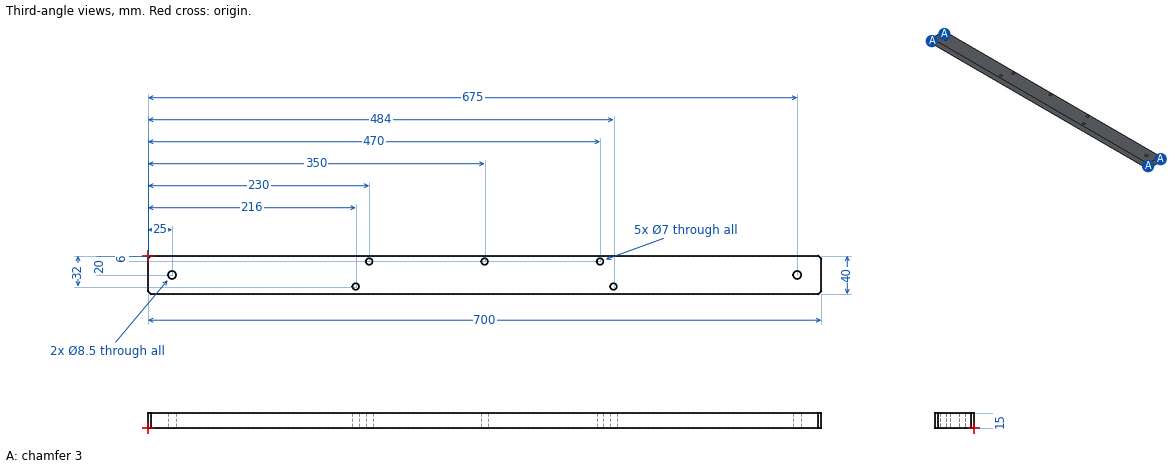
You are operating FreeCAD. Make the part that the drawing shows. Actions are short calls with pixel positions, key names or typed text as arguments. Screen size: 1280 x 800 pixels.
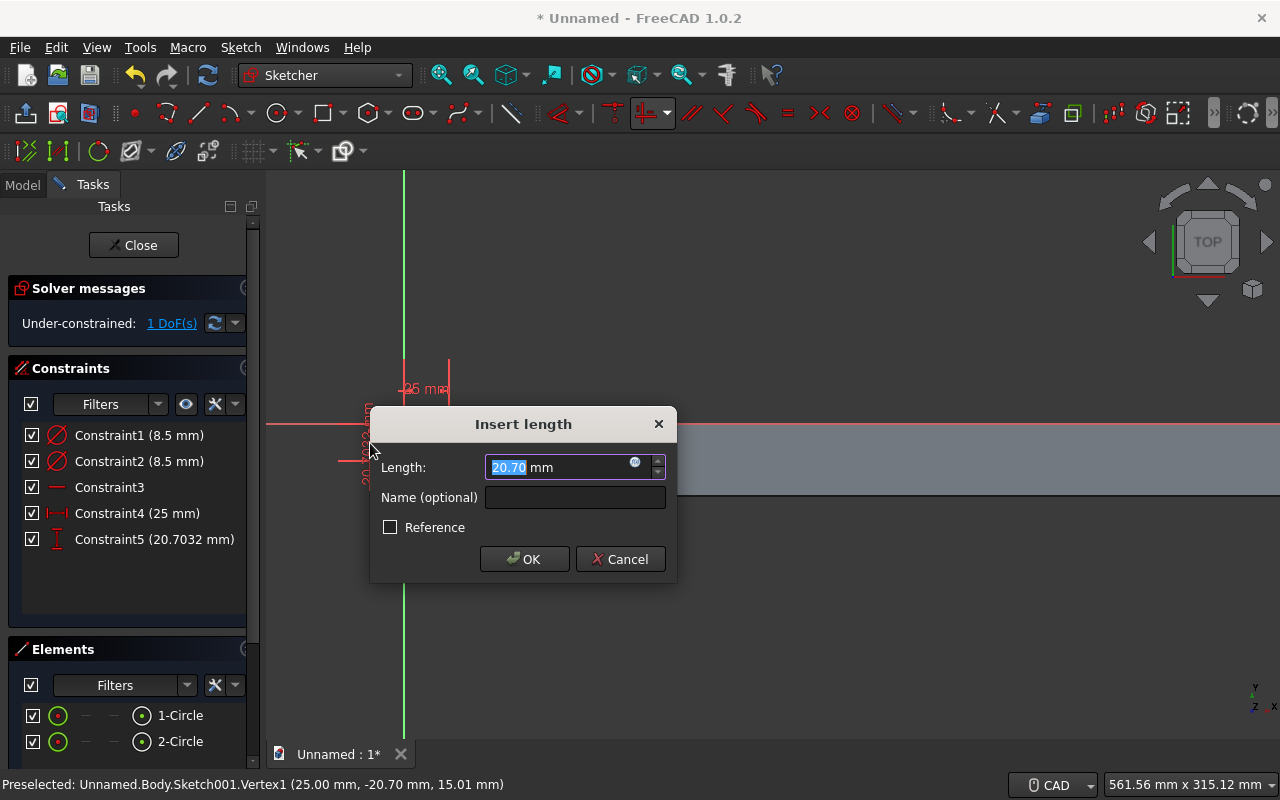
text(20)
key(Return)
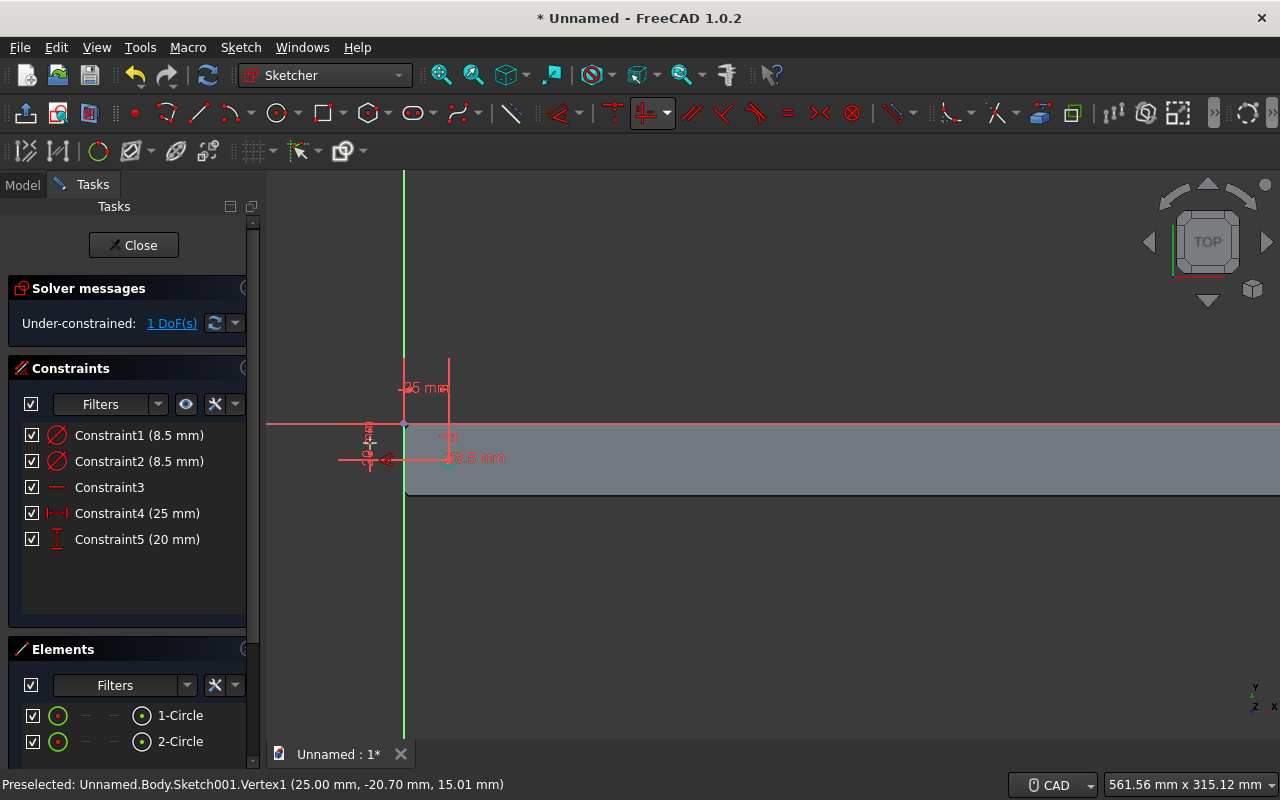
scroll(450, 462, down, 4)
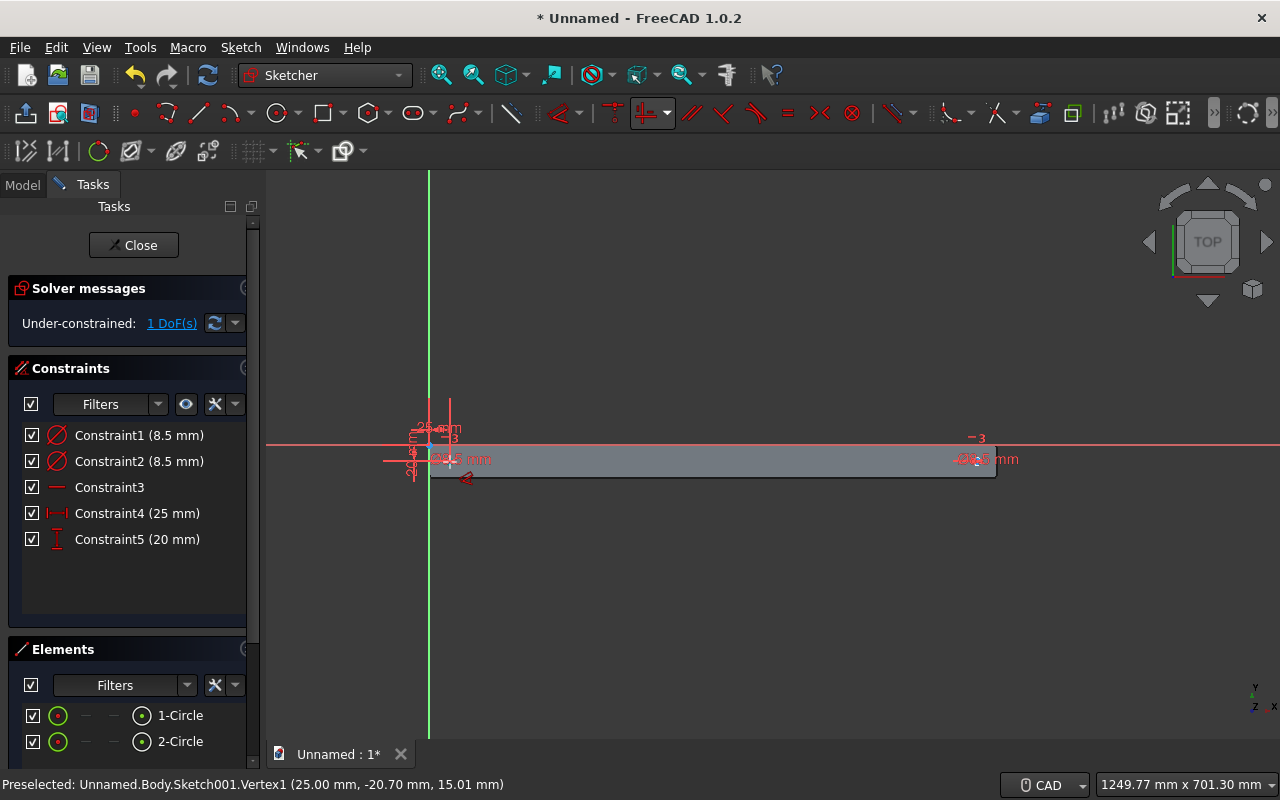
click(977, 461)
click(703, 411)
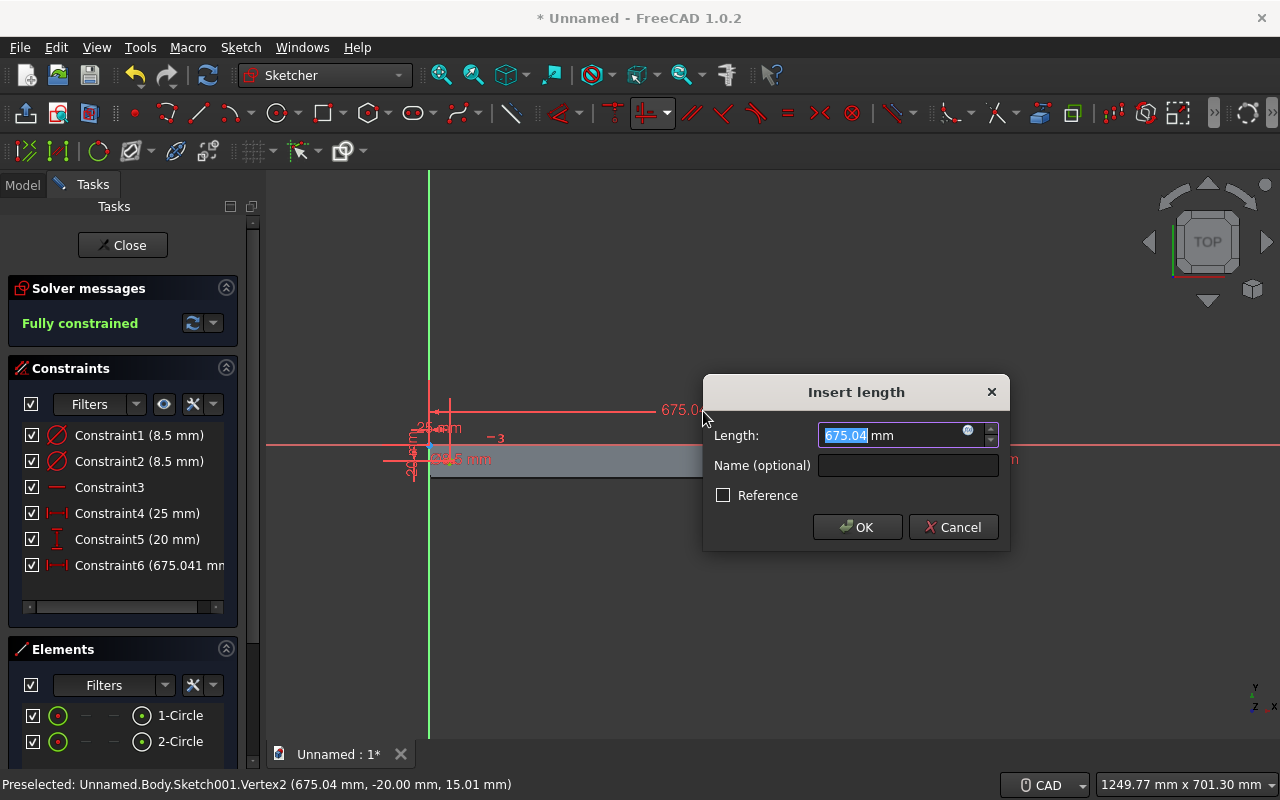
text(675)
key(Return)
key(Escape)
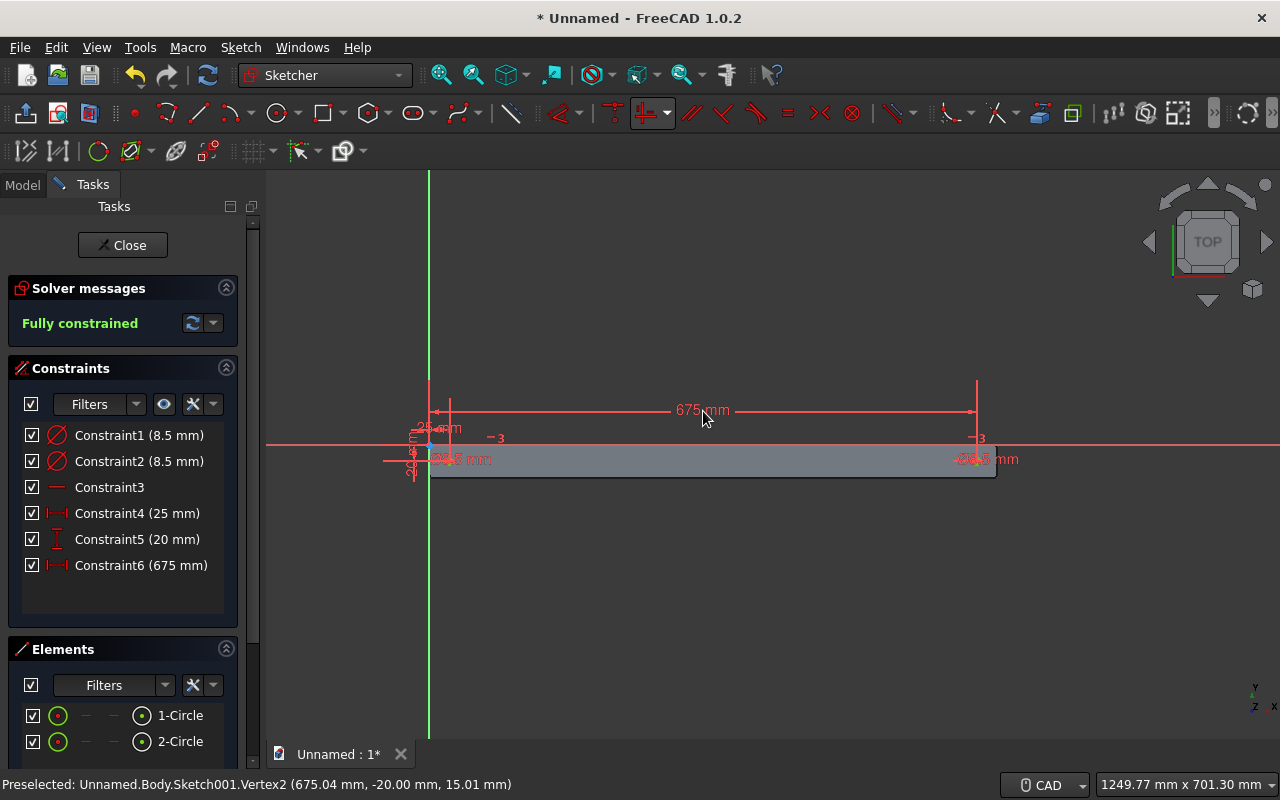
click(123, 245)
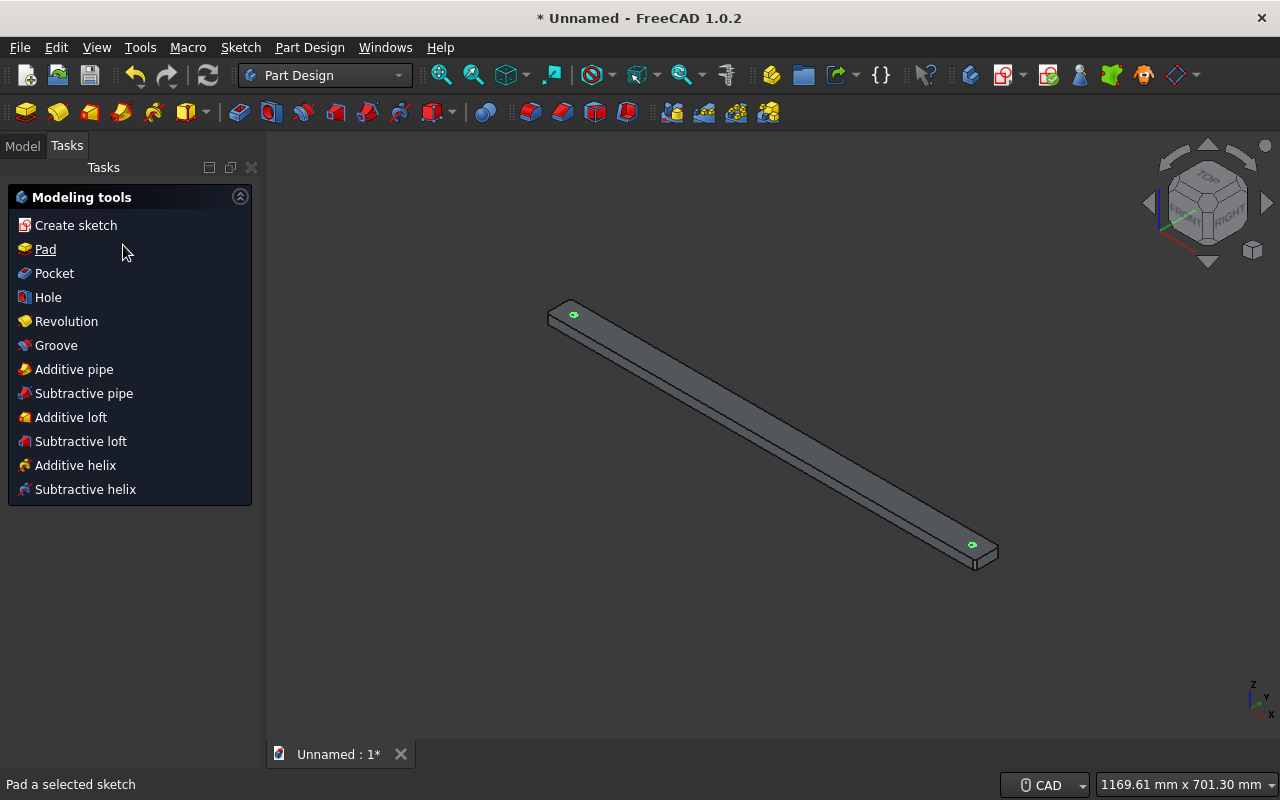
click(272, 112)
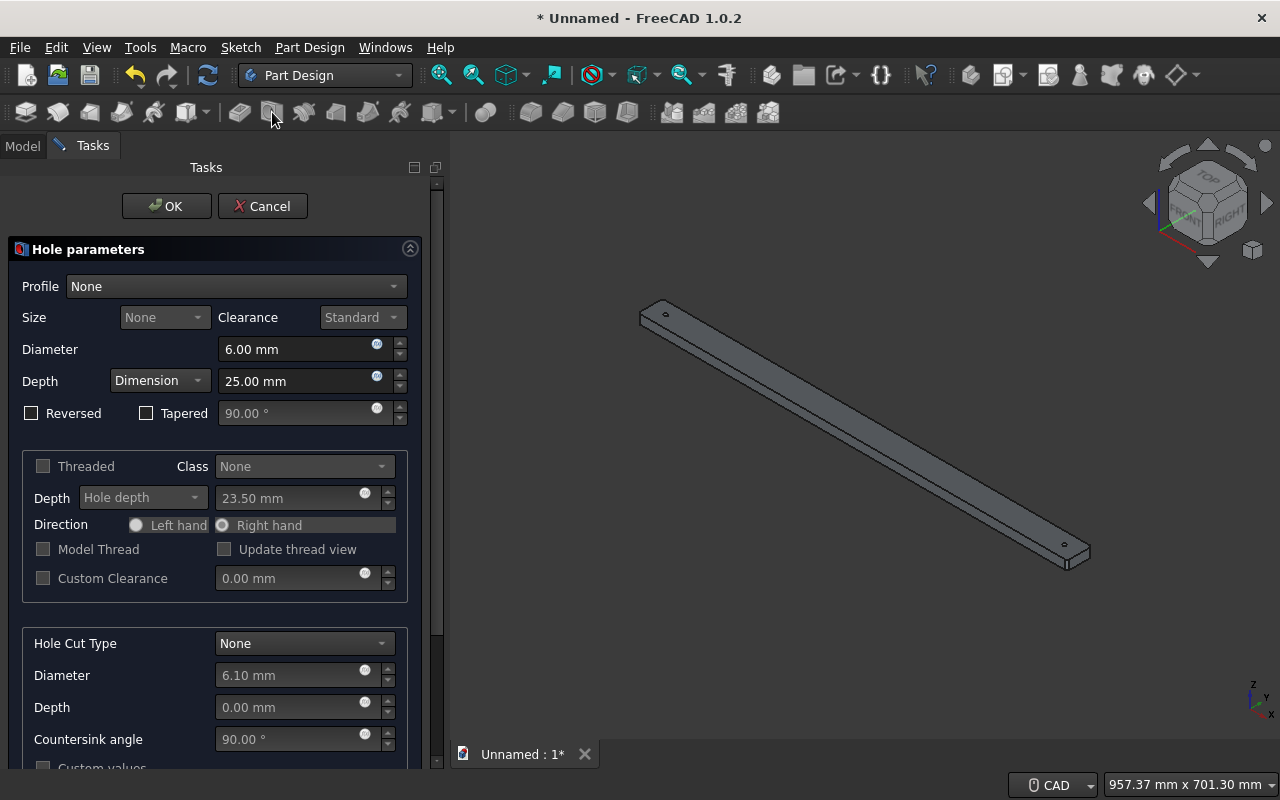
triple_click(305, 349)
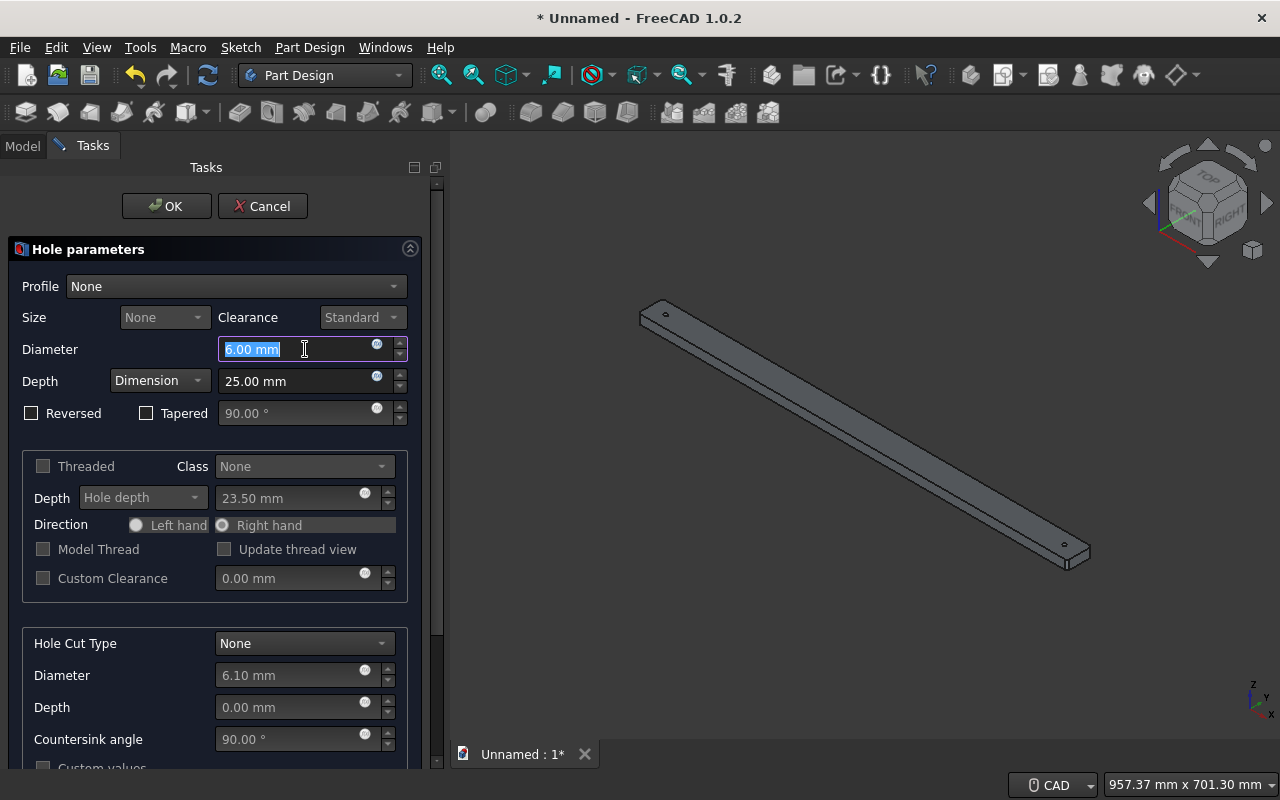
text(8.5)
key(Tab)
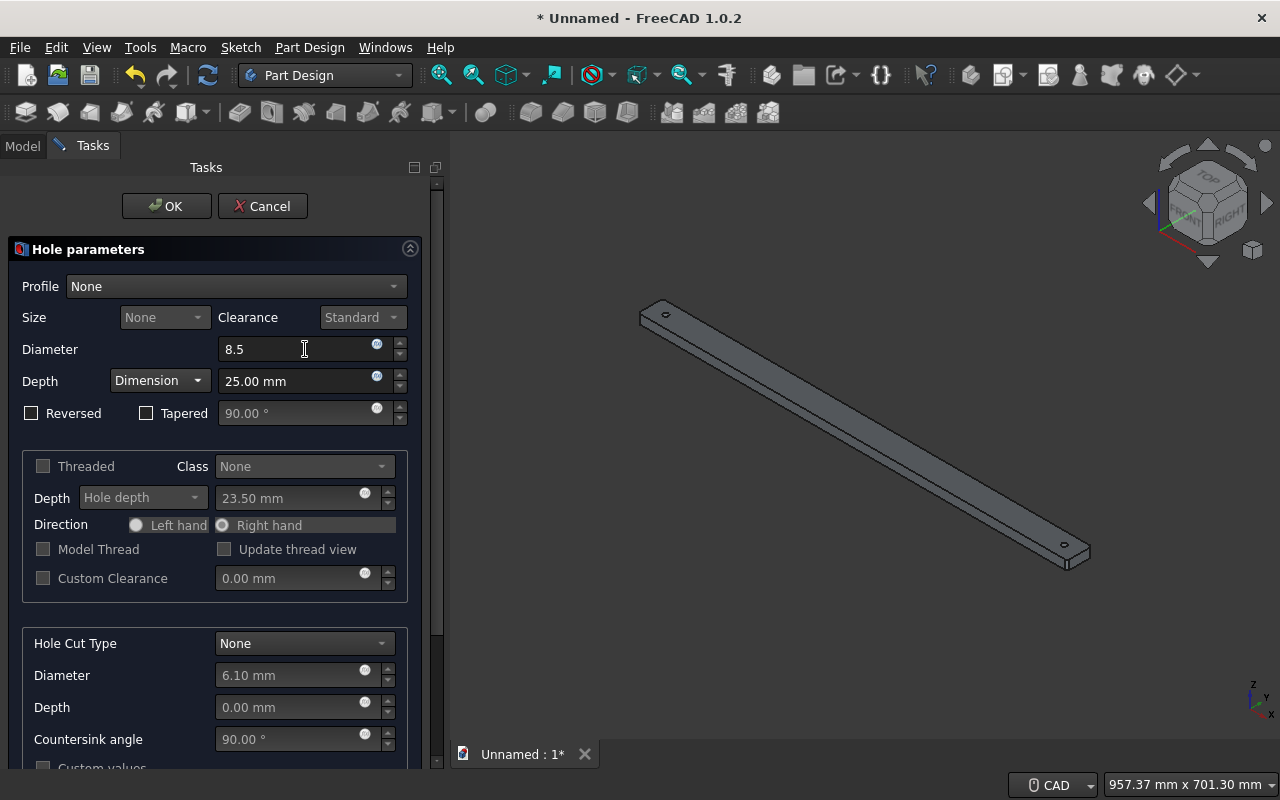
click(161, 380)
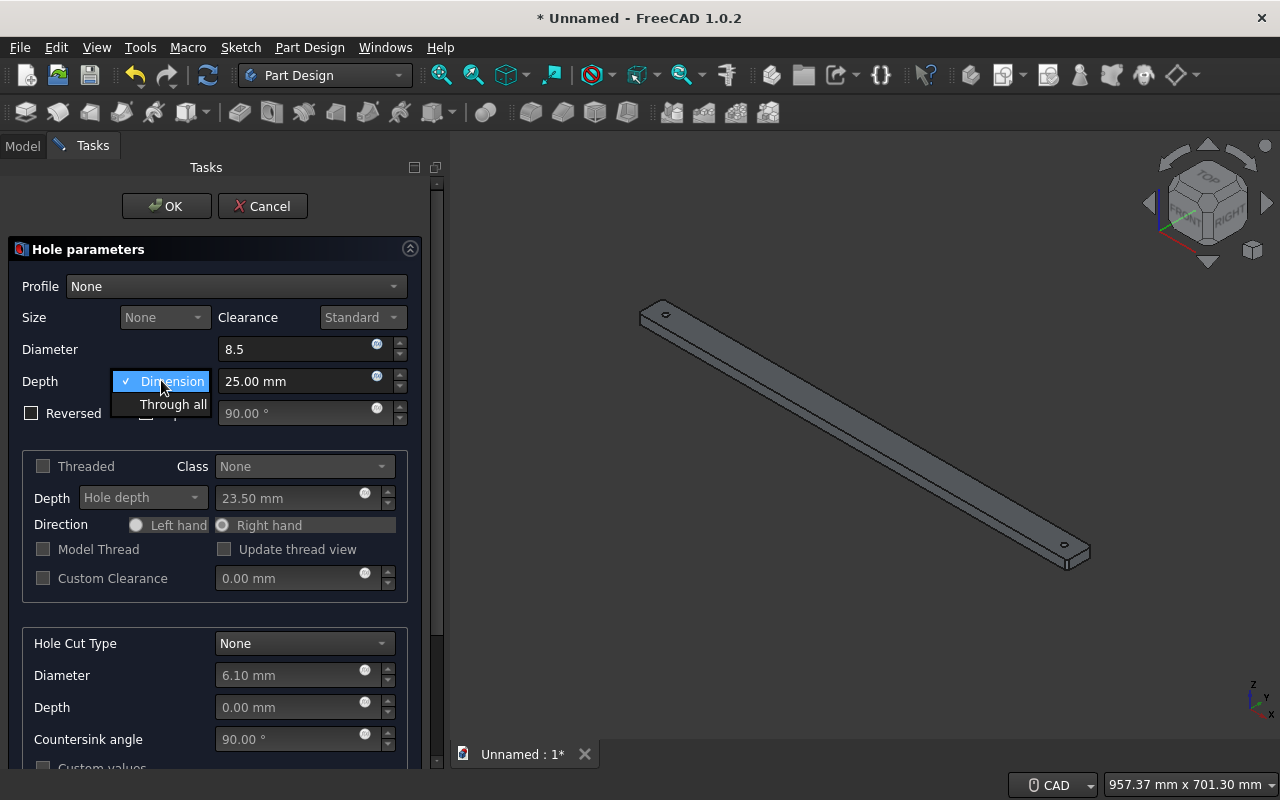
click(160, 404)